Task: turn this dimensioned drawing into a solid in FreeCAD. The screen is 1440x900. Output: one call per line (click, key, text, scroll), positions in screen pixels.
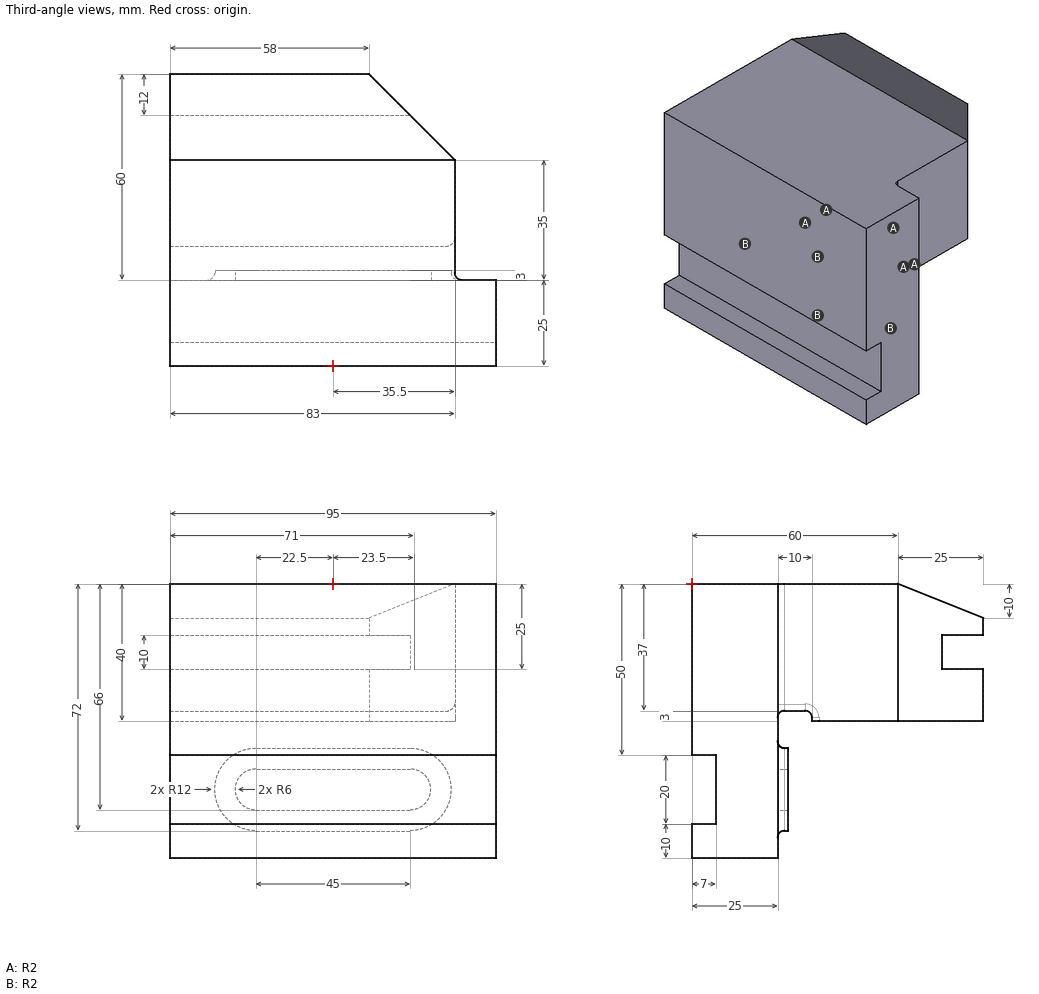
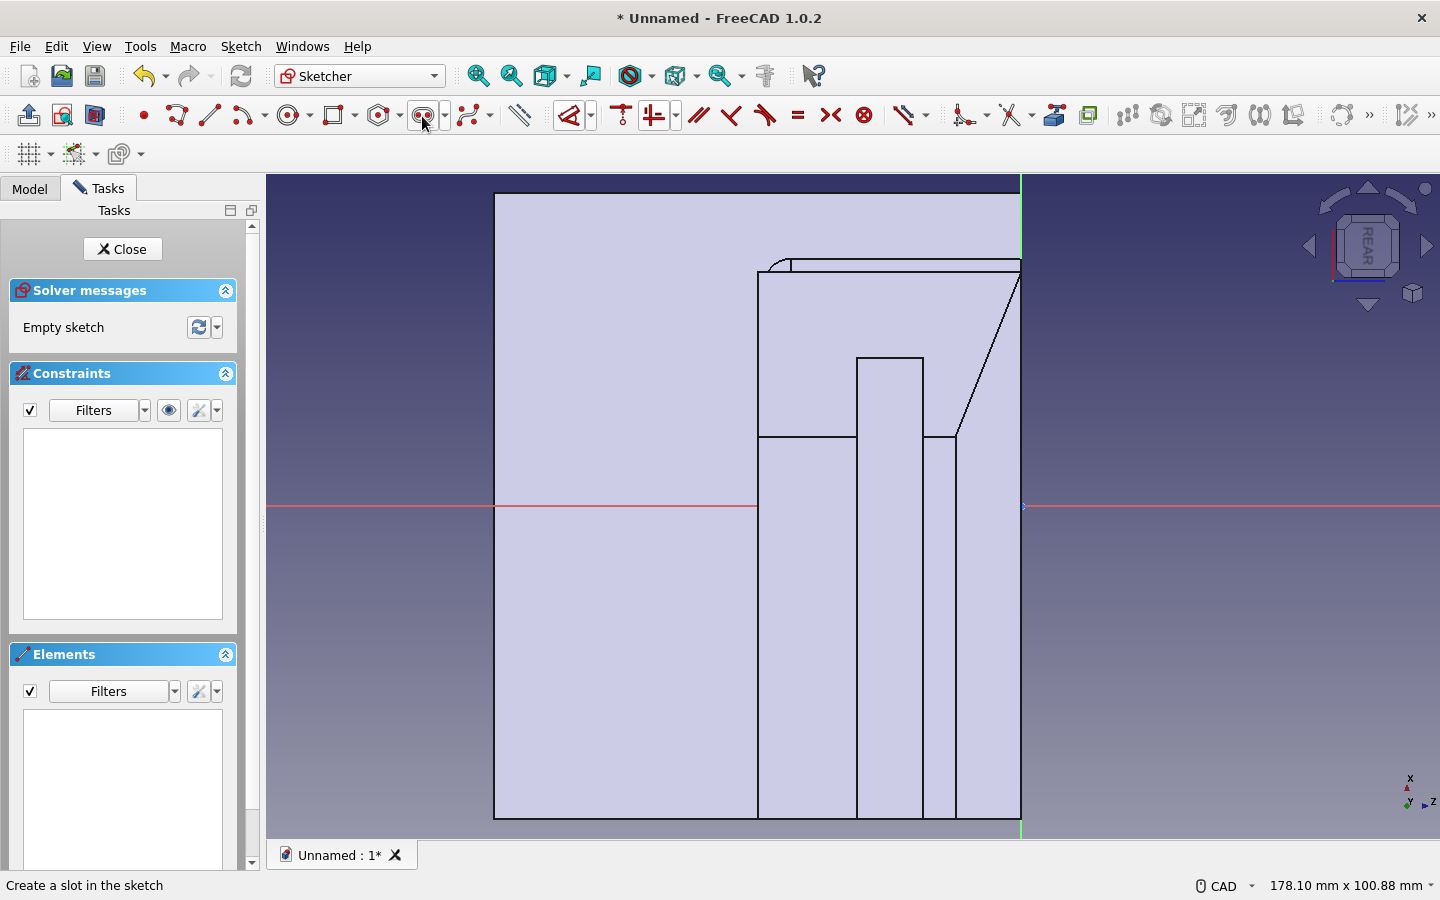
click(626, 654)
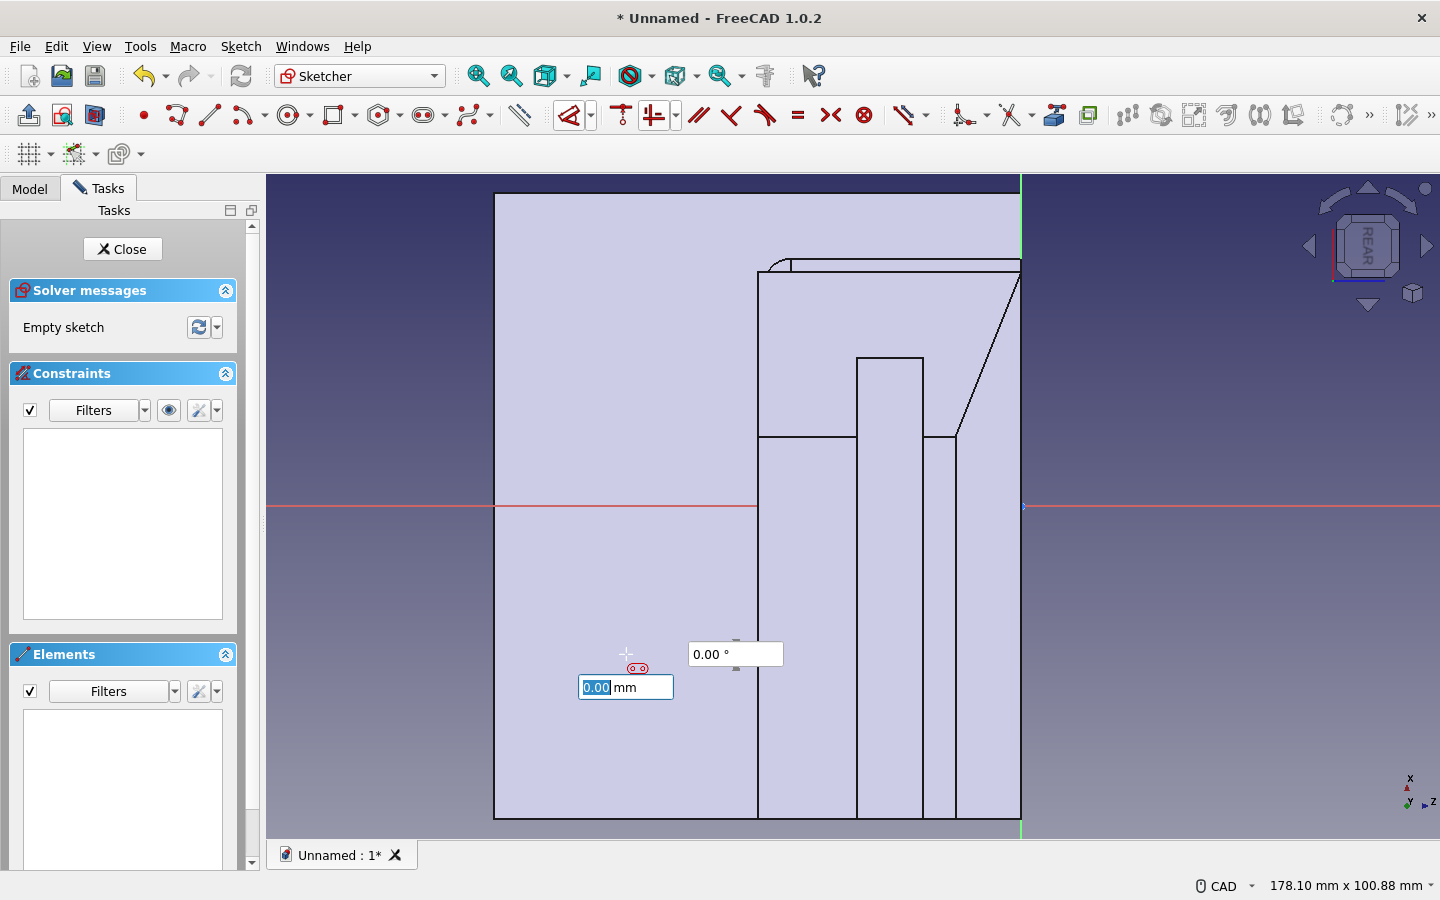
click(626, 358)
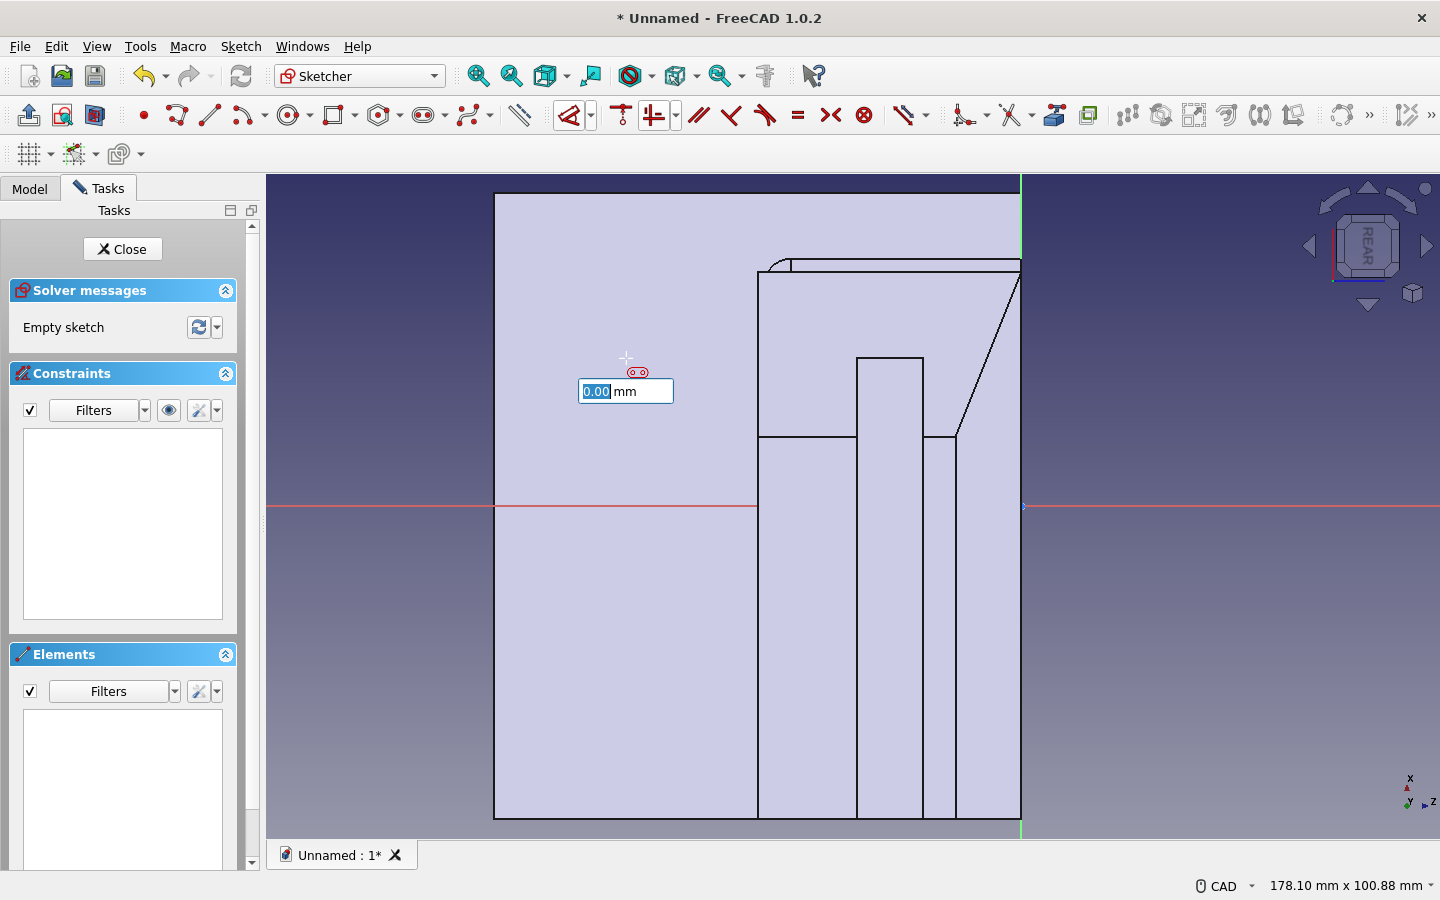
click(547, 462)
key(Escape)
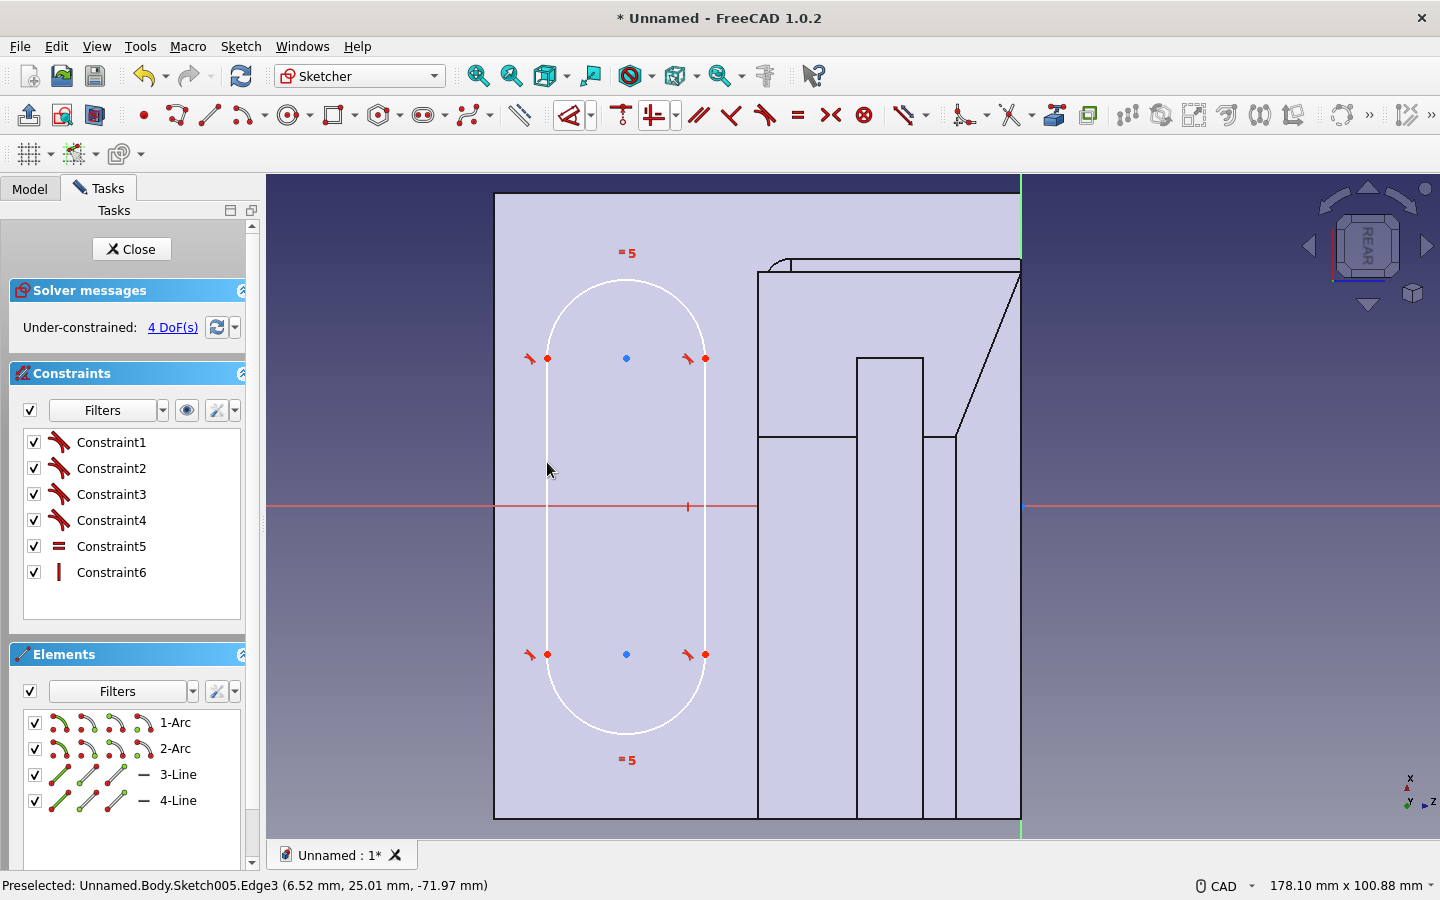
click(580, 719)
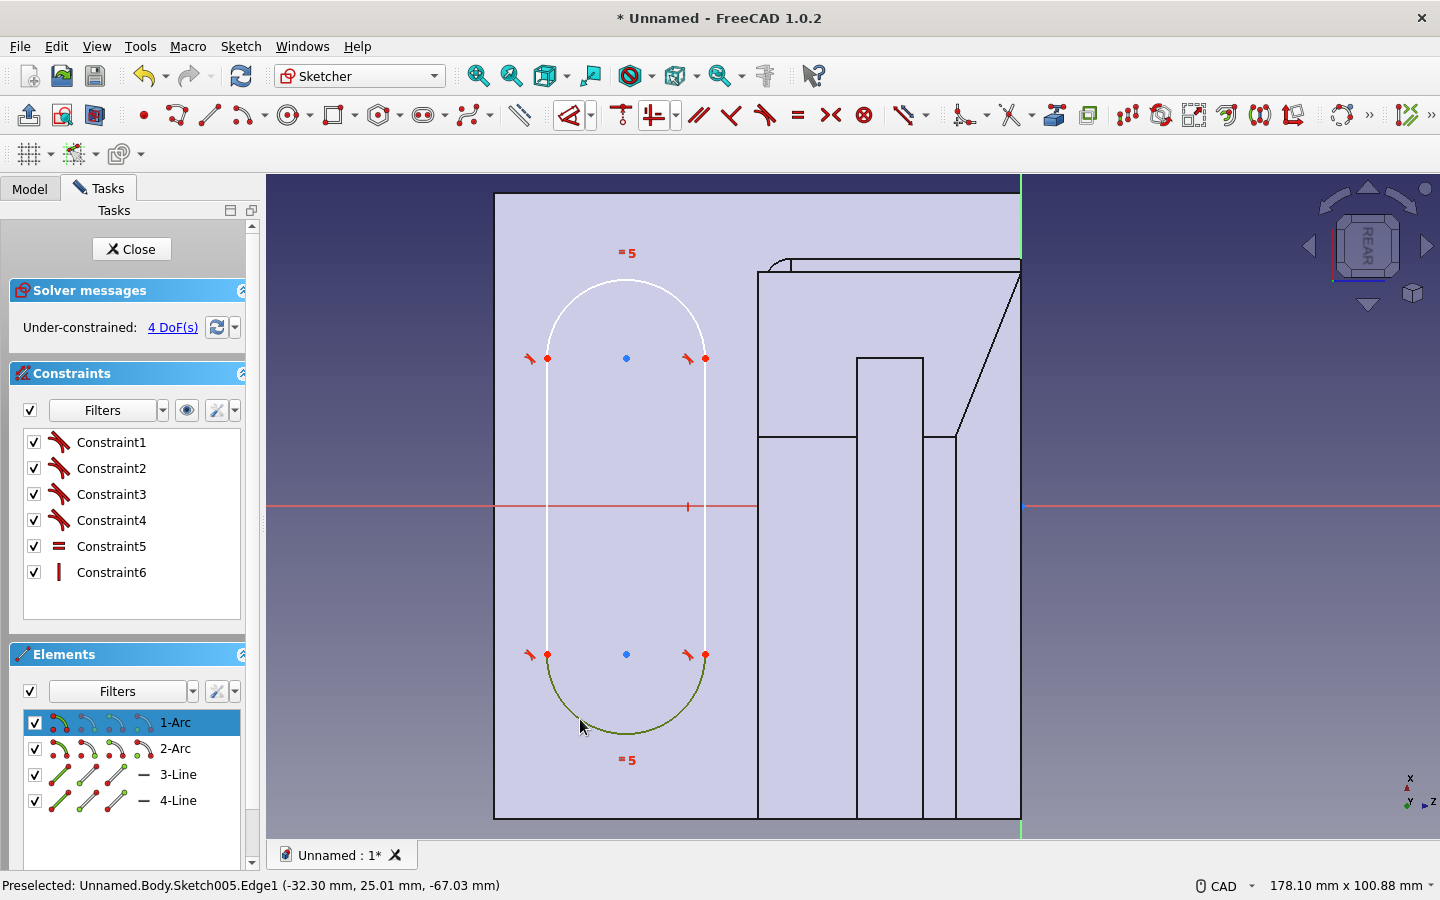
key(k)
key(r)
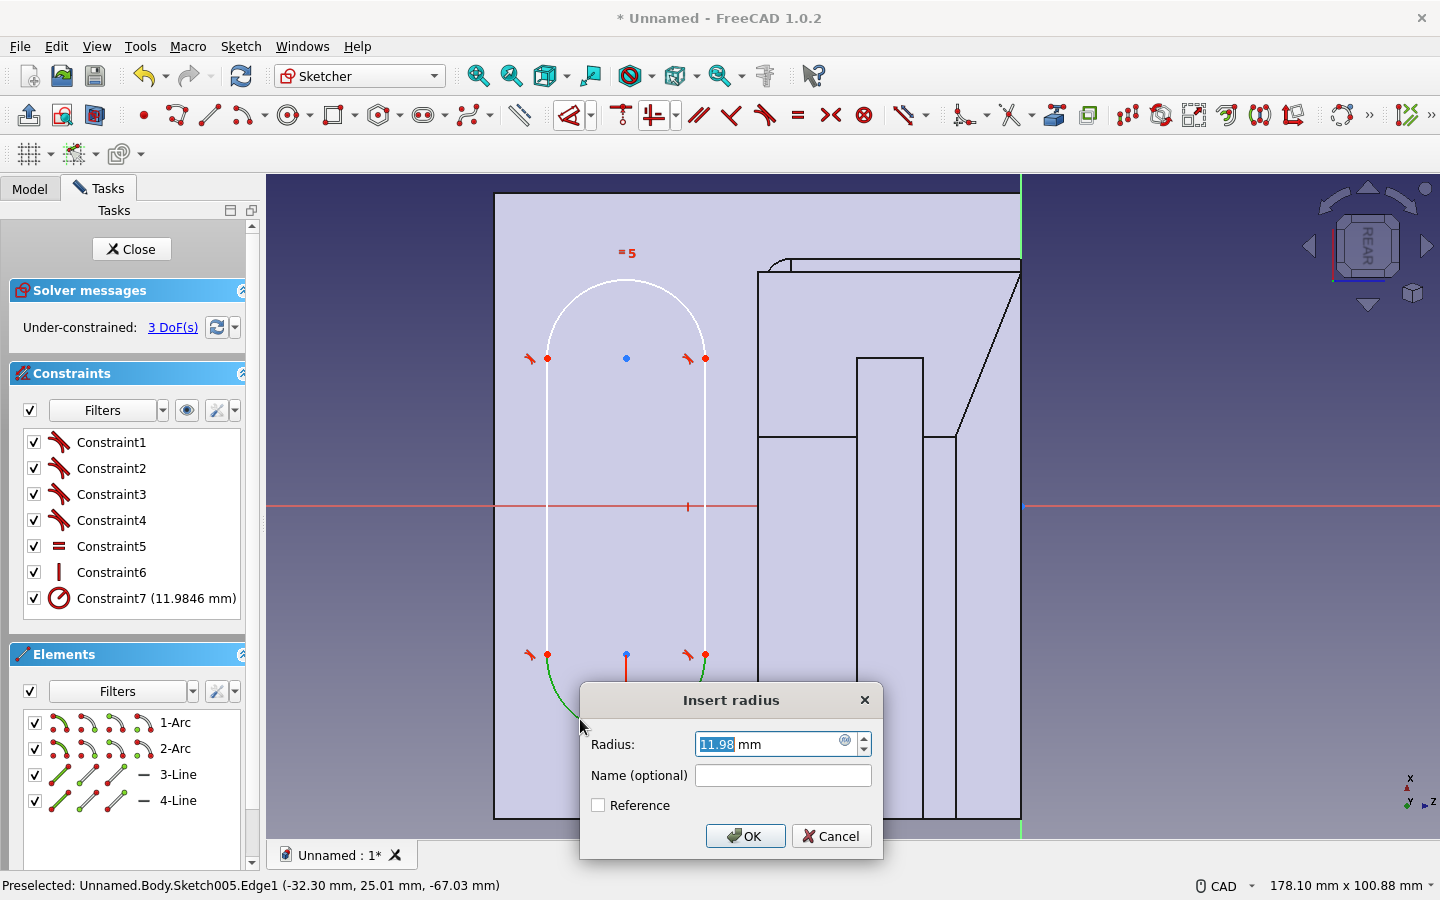
text(12)
key(Return)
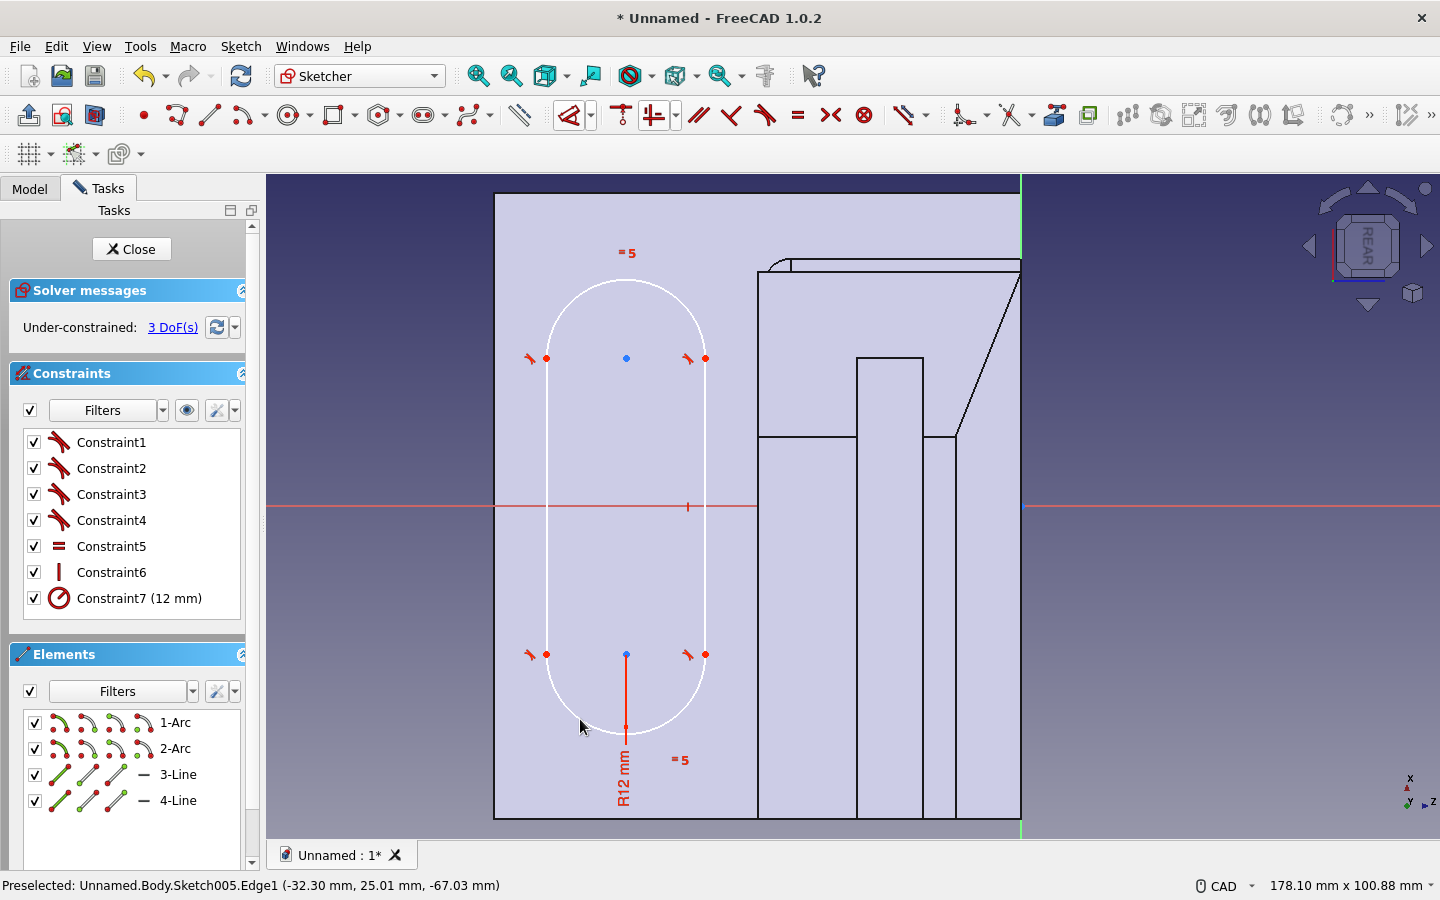
click(547, 566)